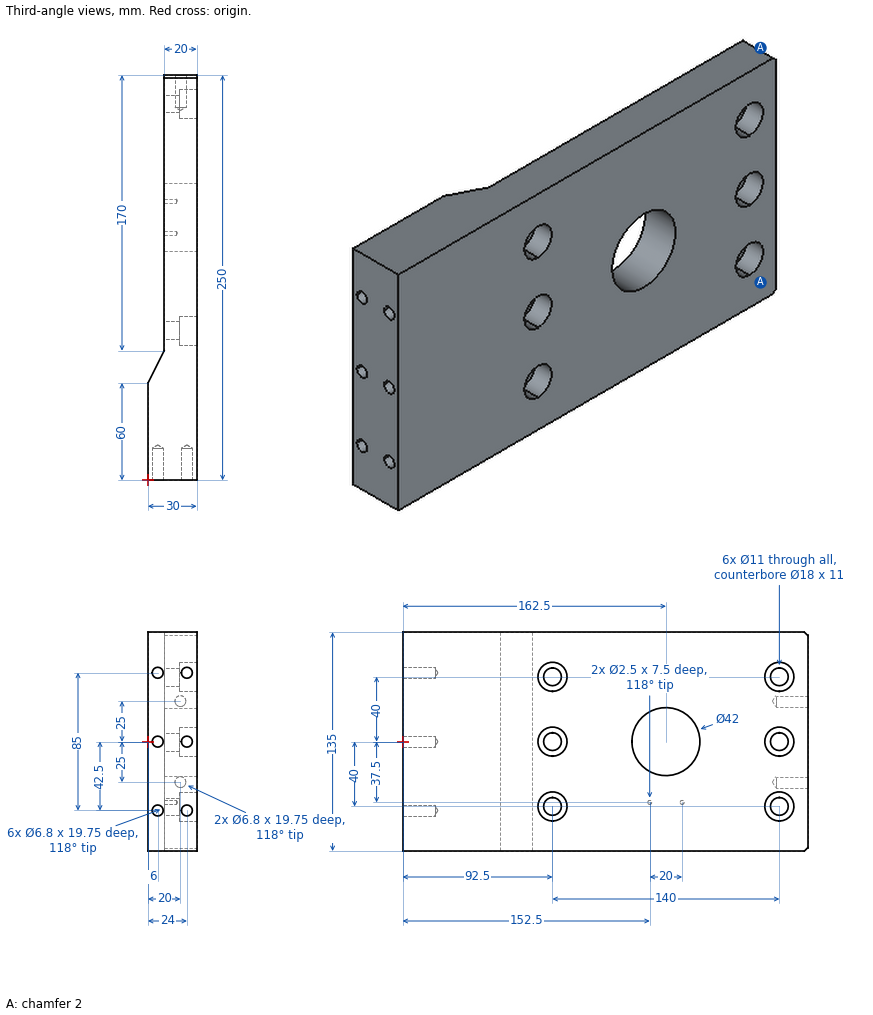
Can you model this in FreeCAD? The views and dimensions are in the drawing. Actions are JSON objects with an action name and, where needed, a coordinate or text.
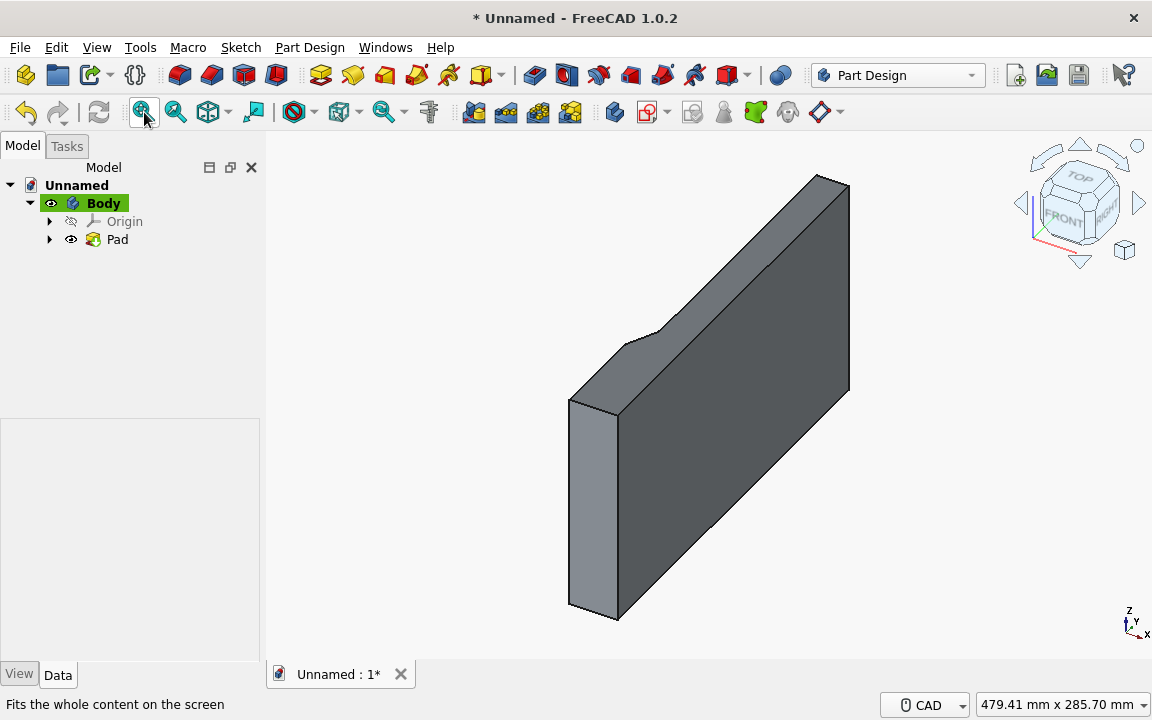
{"action": "left_click", "coordinate": [593, 450]}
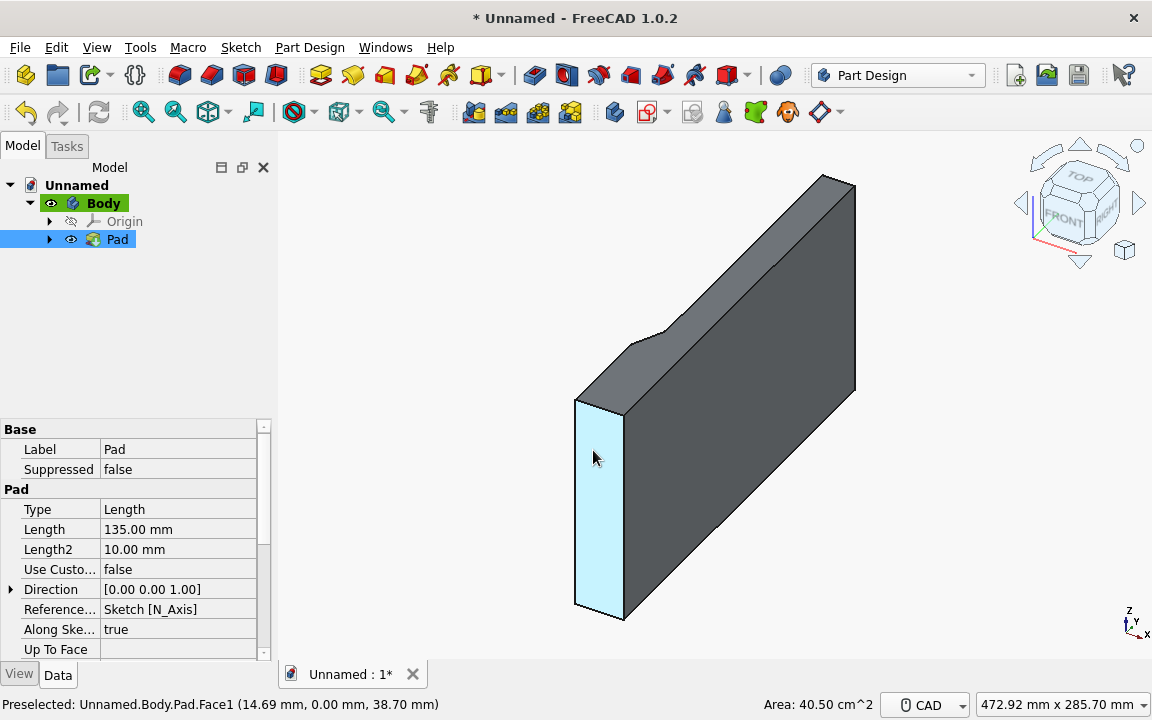
{"action": "left_click", "coordinate": [648, 112]}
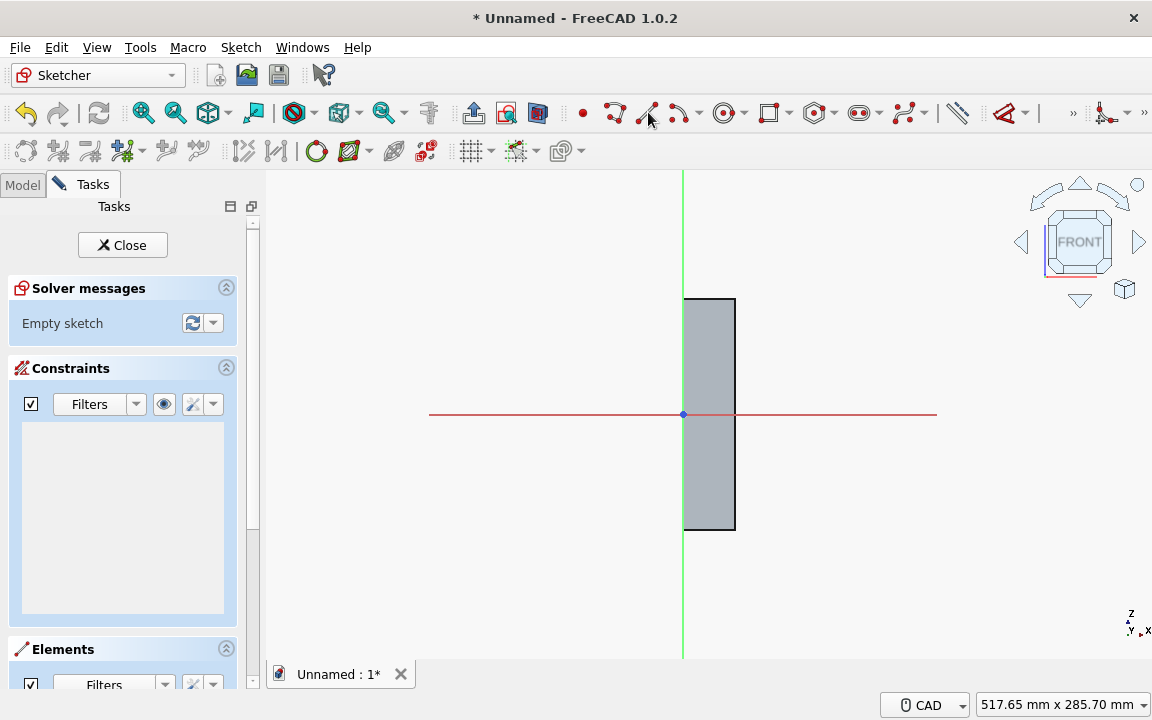
{"action": "scroll", "coordinate": [787, 415], "scroll_direction": "up", "scroll_amount": 3}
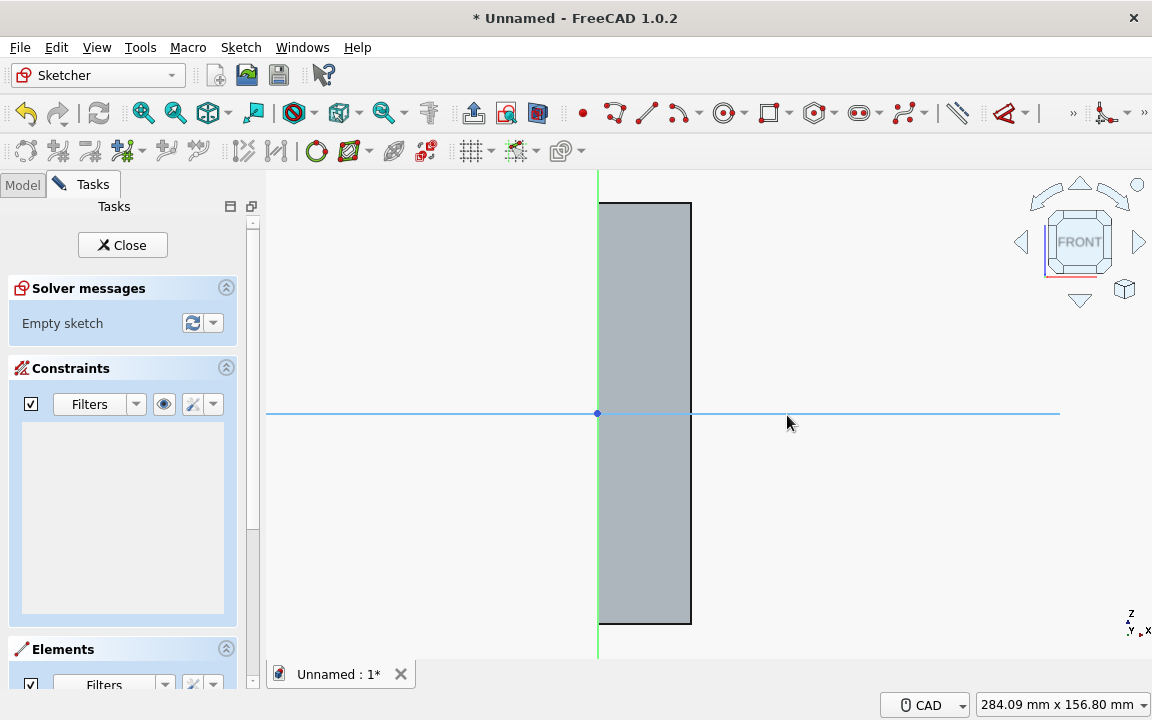
{"action": "left_click", "coordinate": [724, 114]}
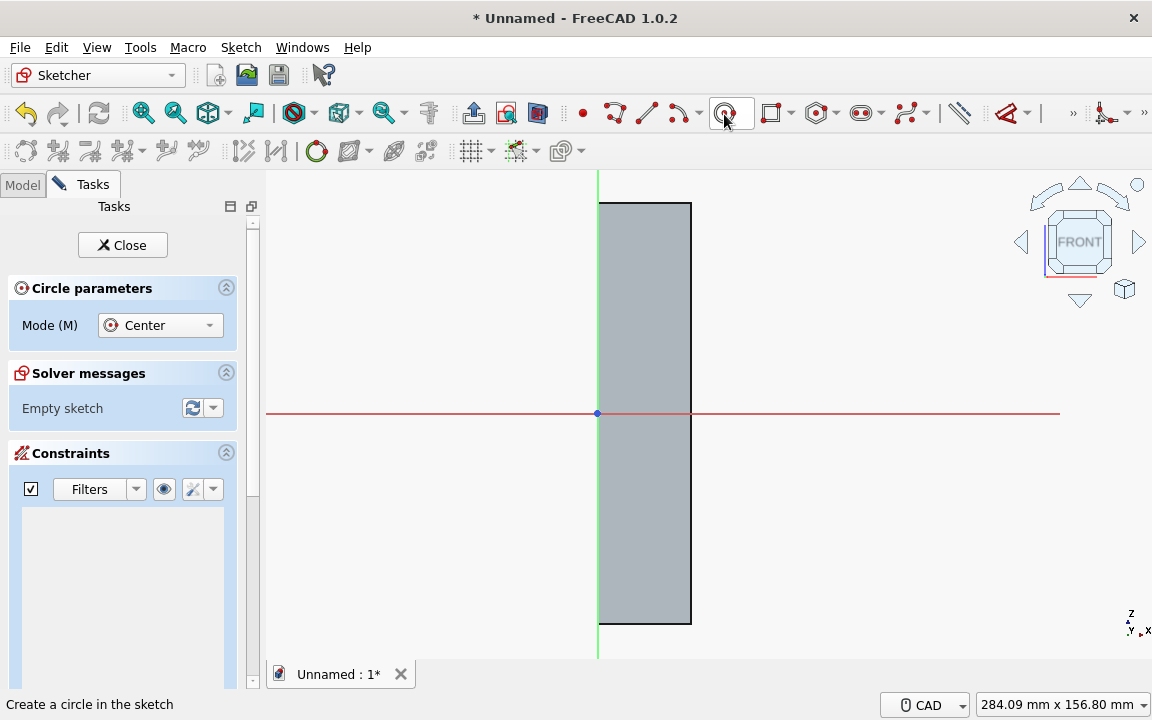
{"action": "scroll", "coordinate": [616, 546], "scroll_direction": "up", "scroll_amount": 4}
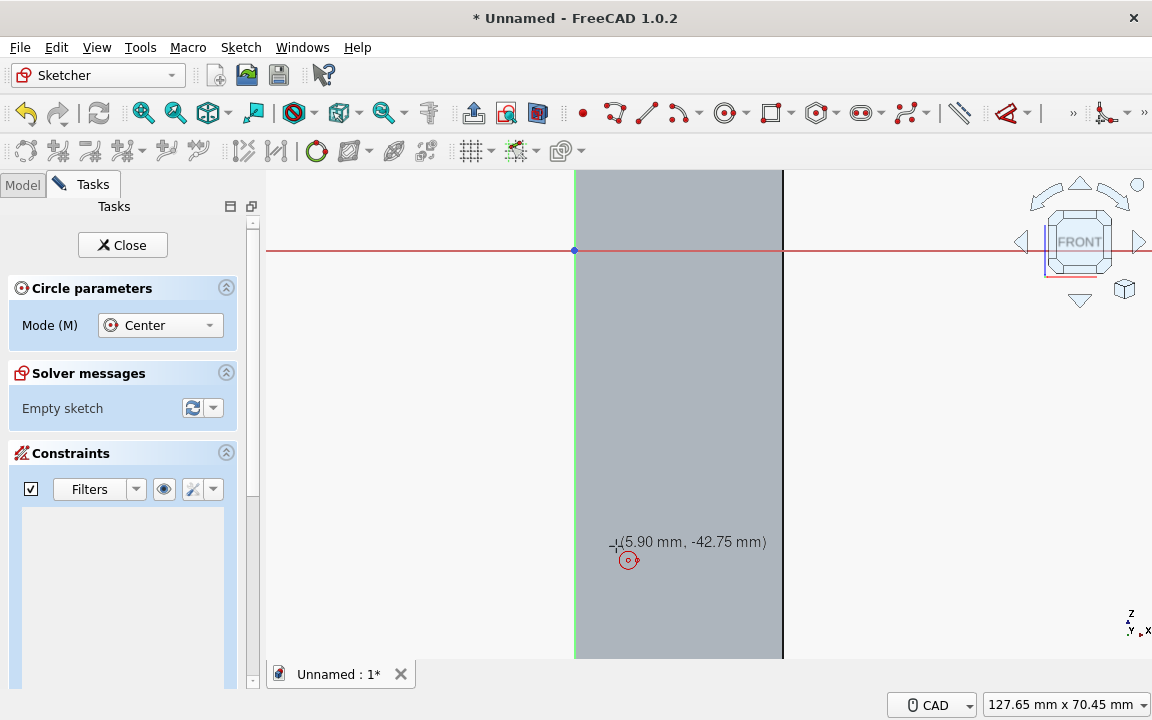
{"action": "left_click", "coordinate": [616, 546]}
{"action": "mouse_move", "coordinate": [633, 529]}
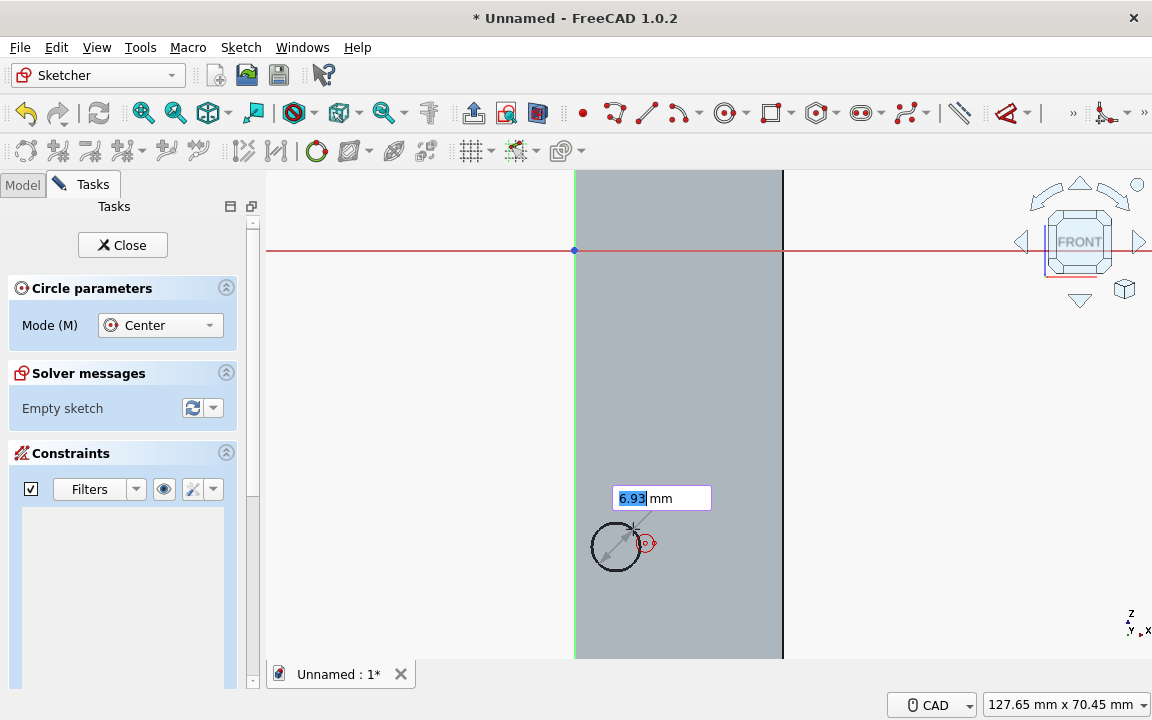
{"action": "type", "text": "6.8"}
{"action": "key", "text": "Return"}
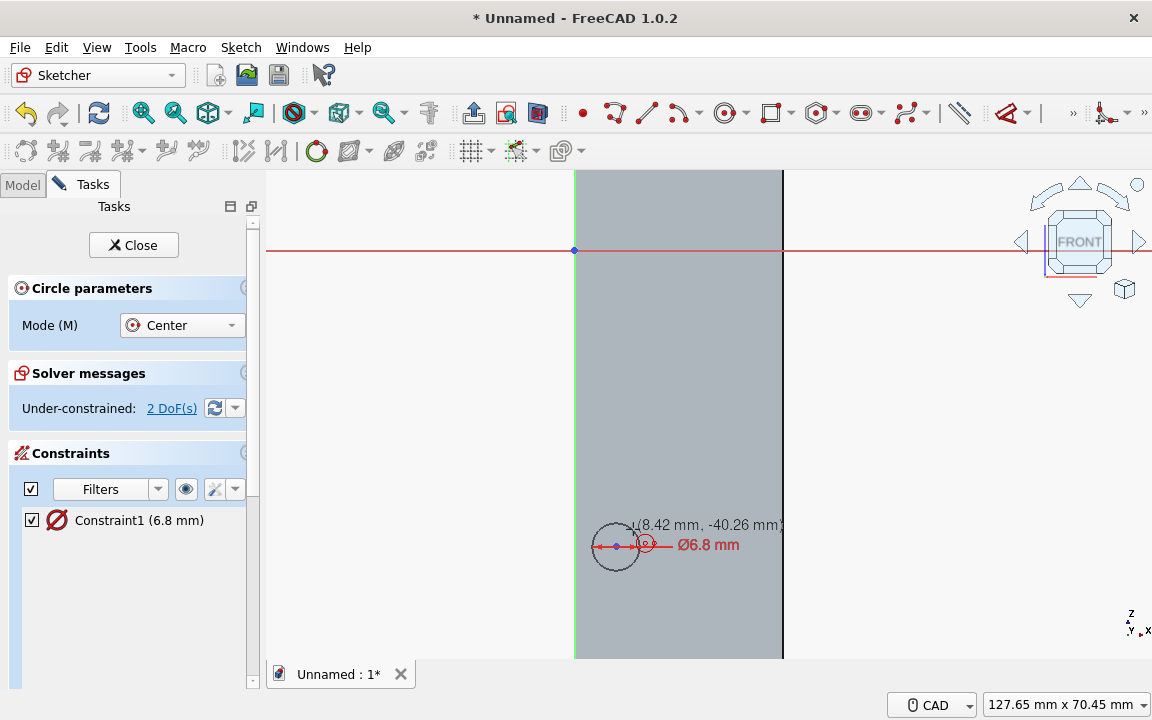
{"action": "left_click", "coordinate": [741, 546]}
{"action": "mouse_move", "coordinate": [758, 529]}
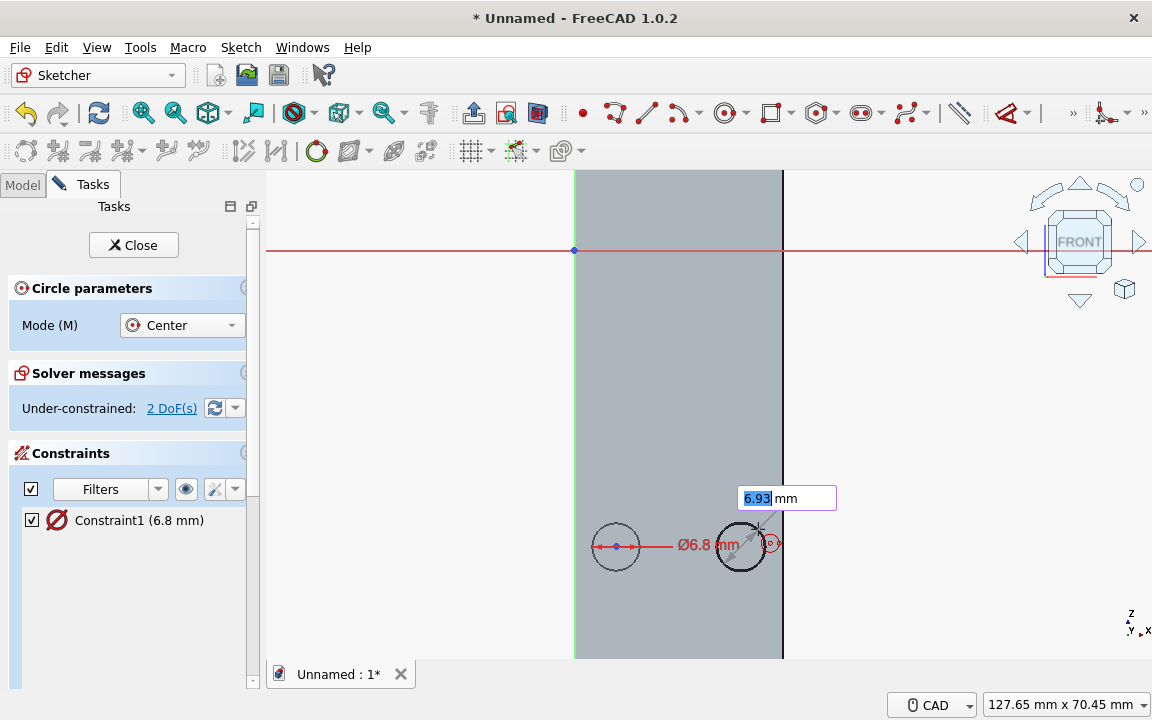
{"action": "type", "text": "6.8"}
{"action": "key", "text": "Return"}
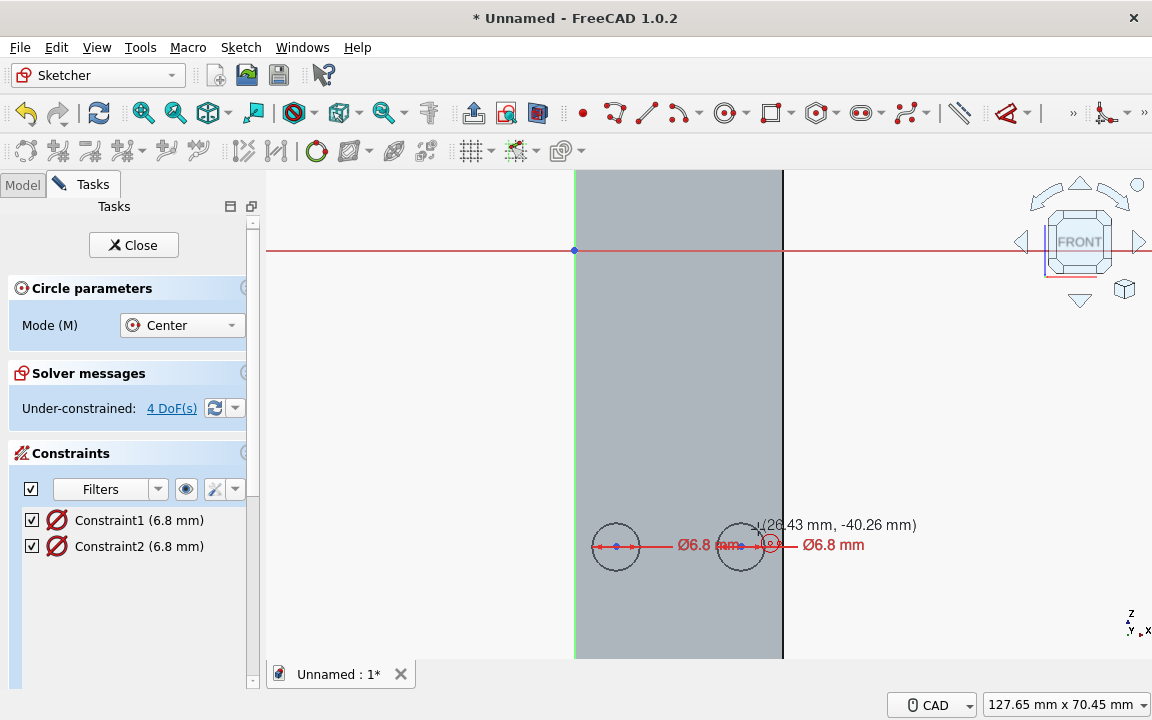
{"action": "left_click", "coordinate": [741, 251]}
{"action": "mouse_move", "coordinate": [758, 234]}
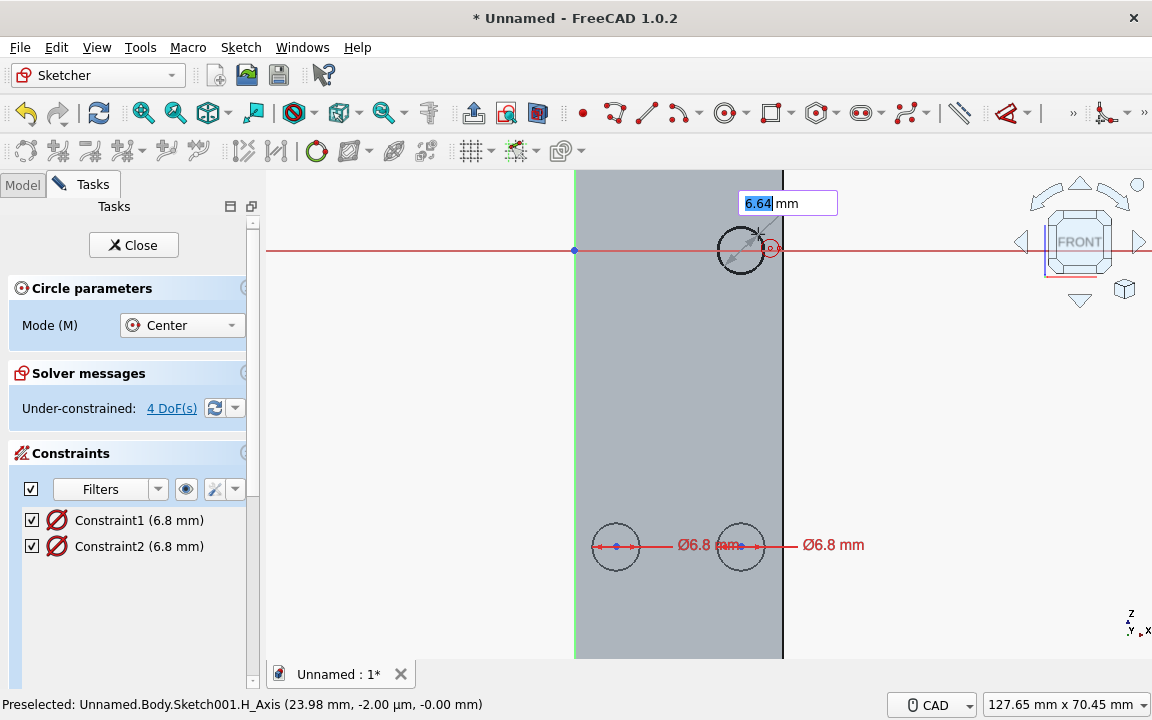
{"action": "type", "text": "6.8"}
{"action": "key", "text": "Return"}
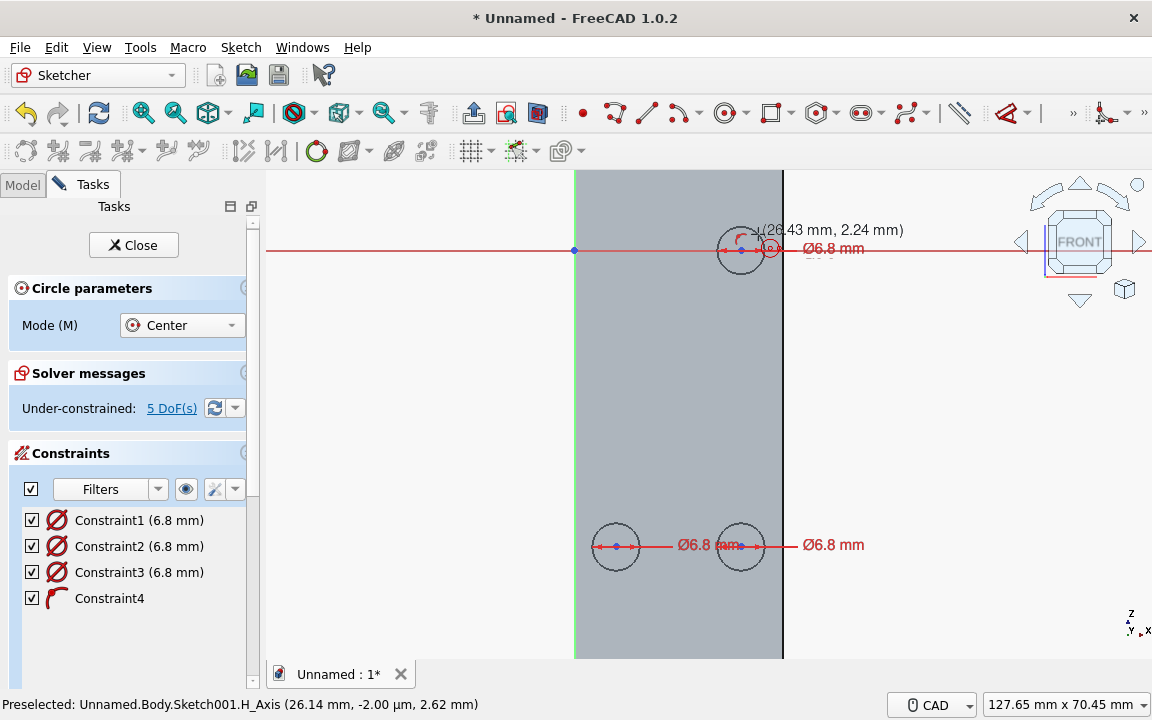
{"action": "left_click", "coordinate": [616, 251]}
{"action": "mouse_move", "coordinate": [633, 234]}